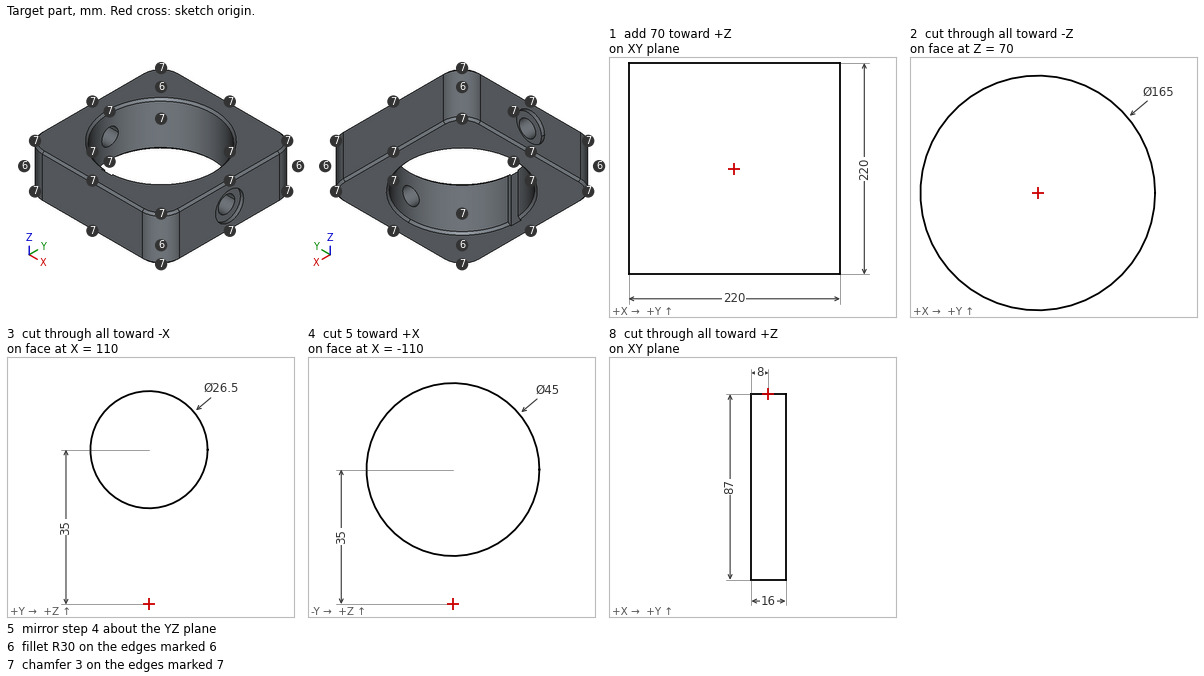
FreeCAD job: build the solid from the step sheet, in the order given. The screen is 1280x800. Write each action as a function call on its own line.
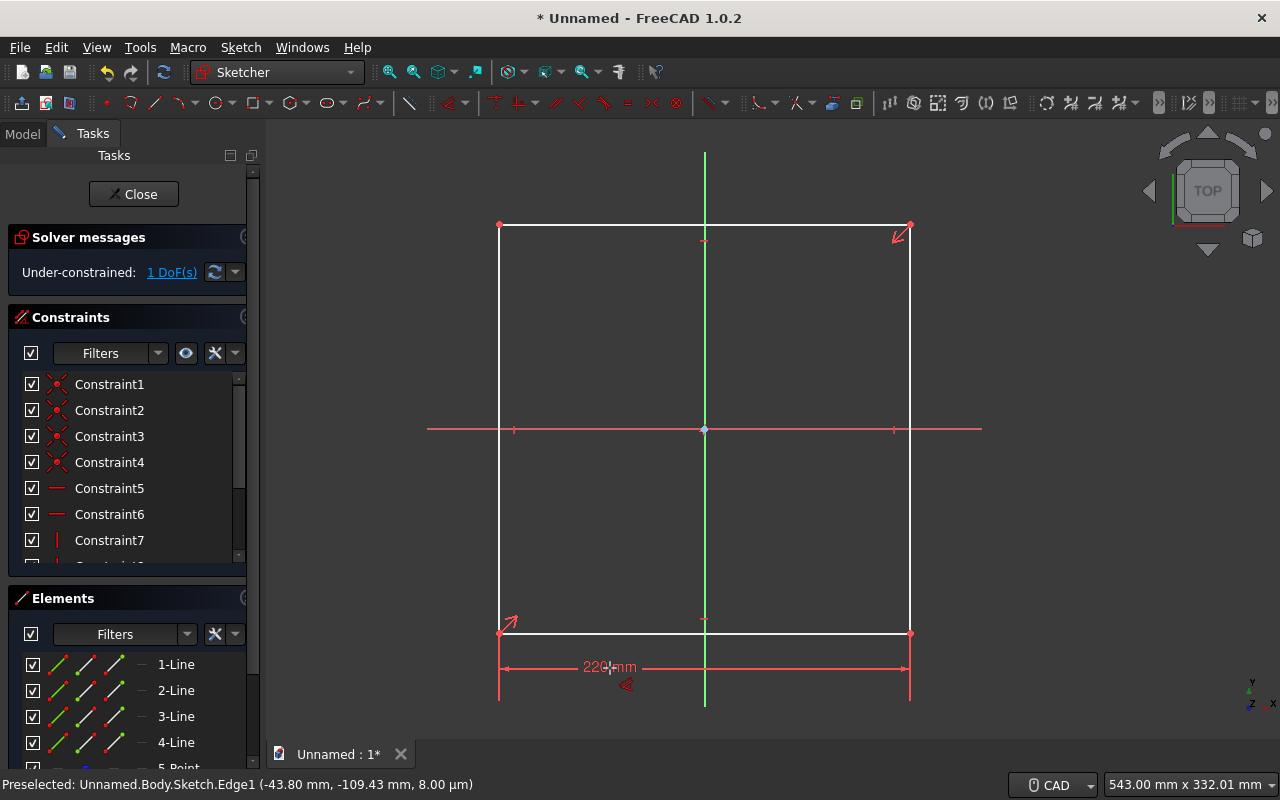
click(910, 511)
click(944, 335)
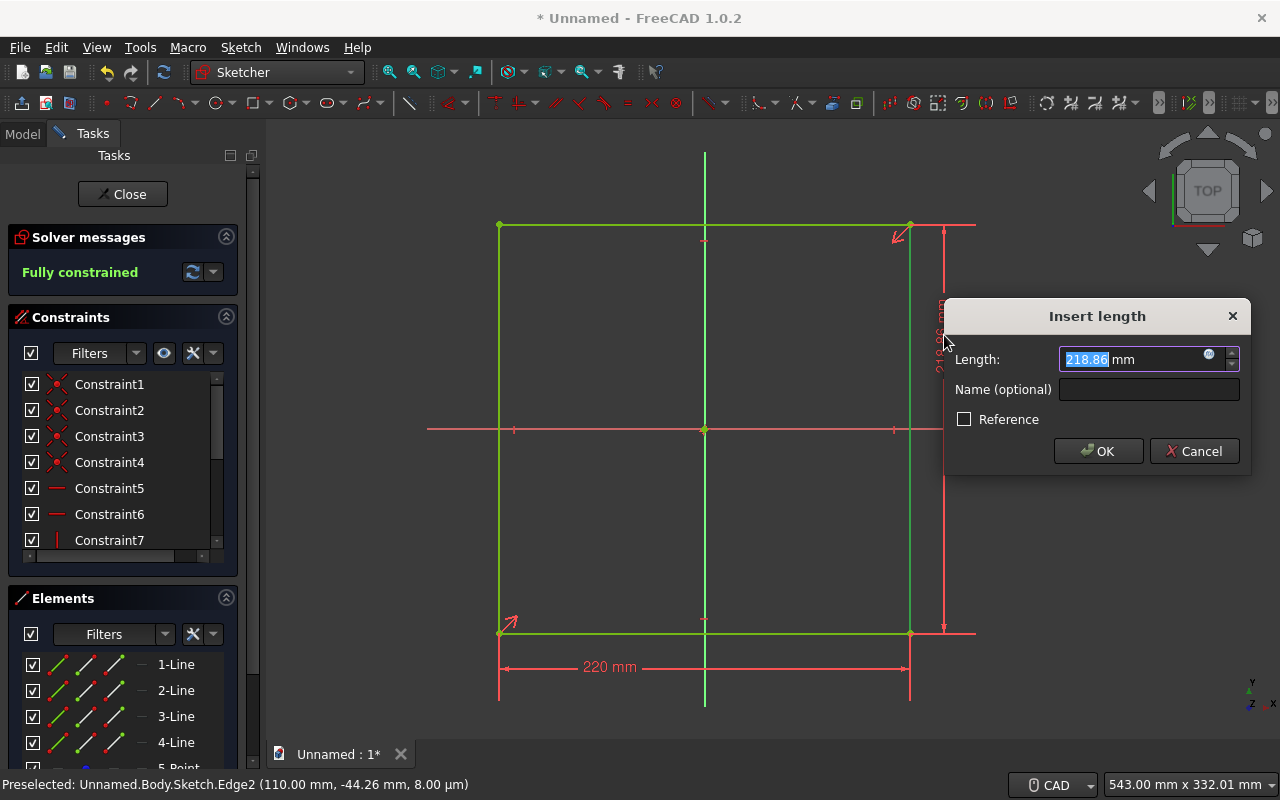
text(220)
key(Return)
key(Escape)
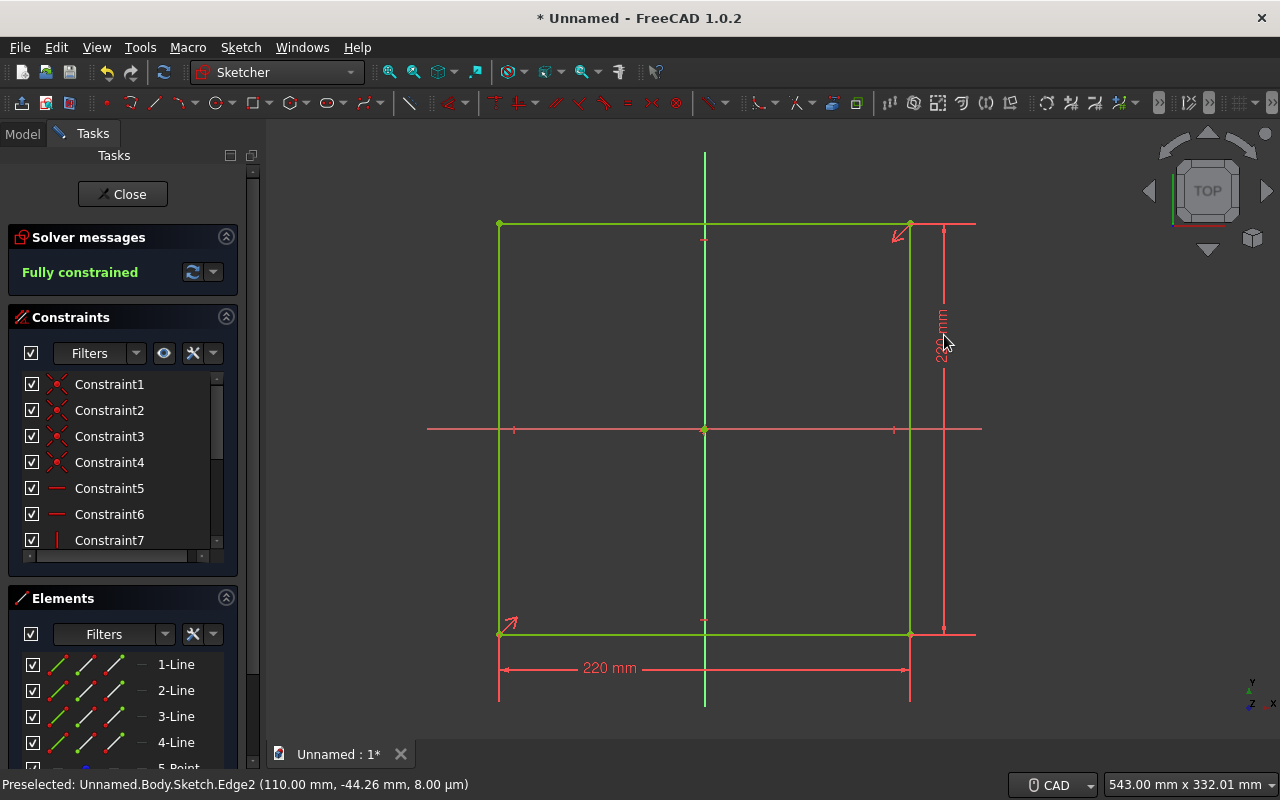
click(123, 194)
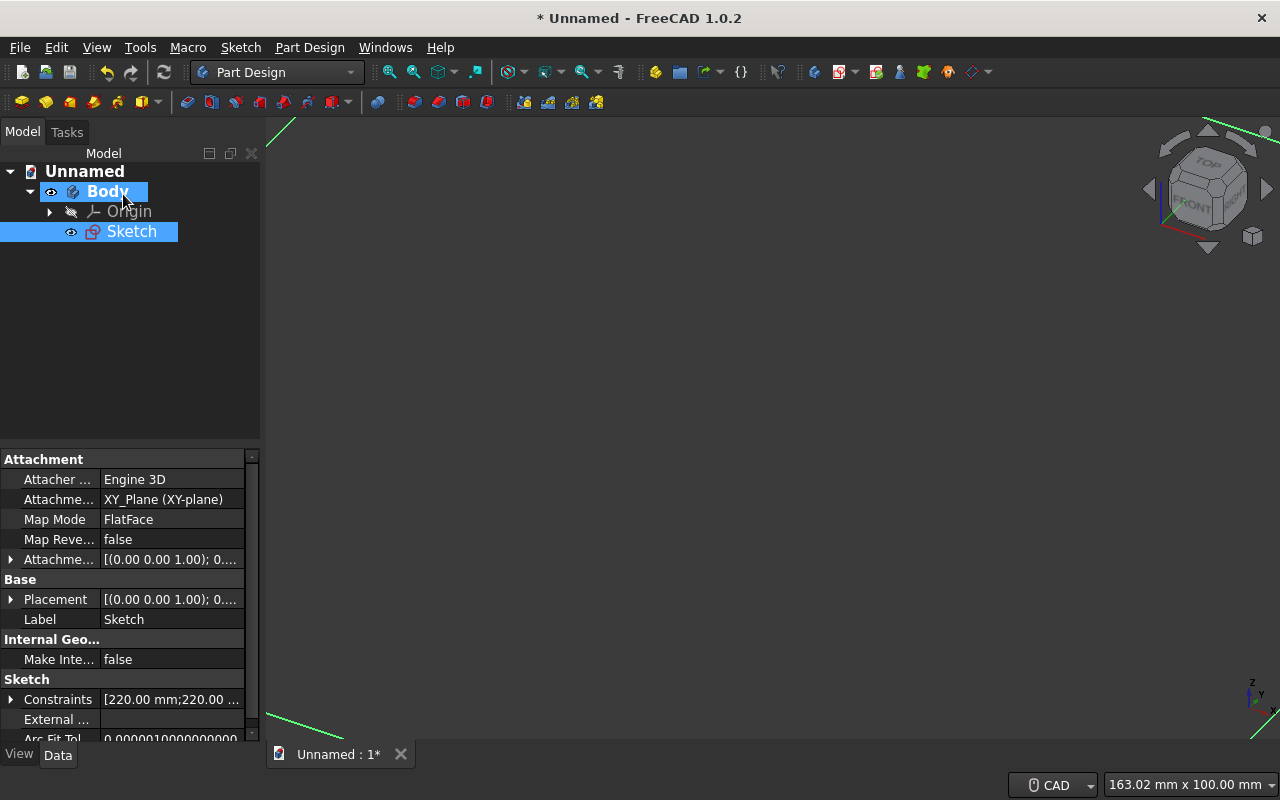
click(22, 102)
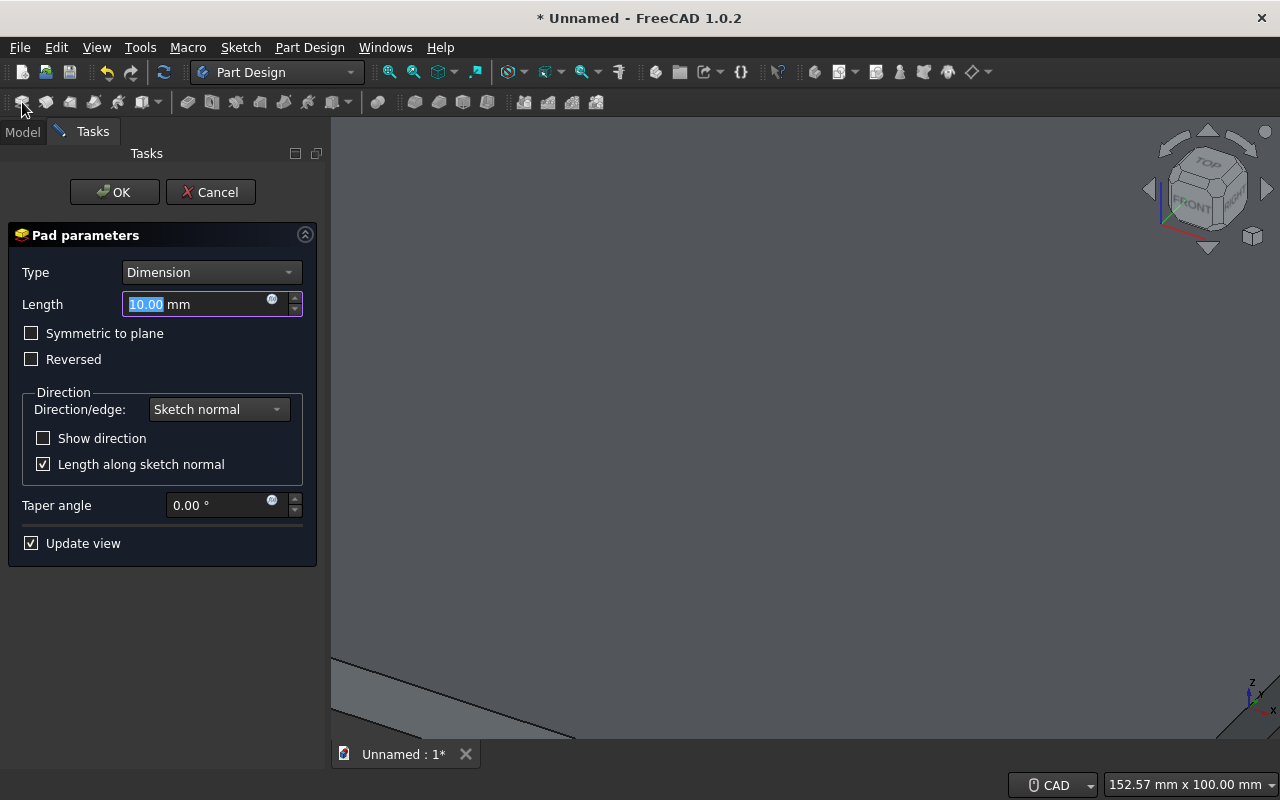
text(70)
key(Tab)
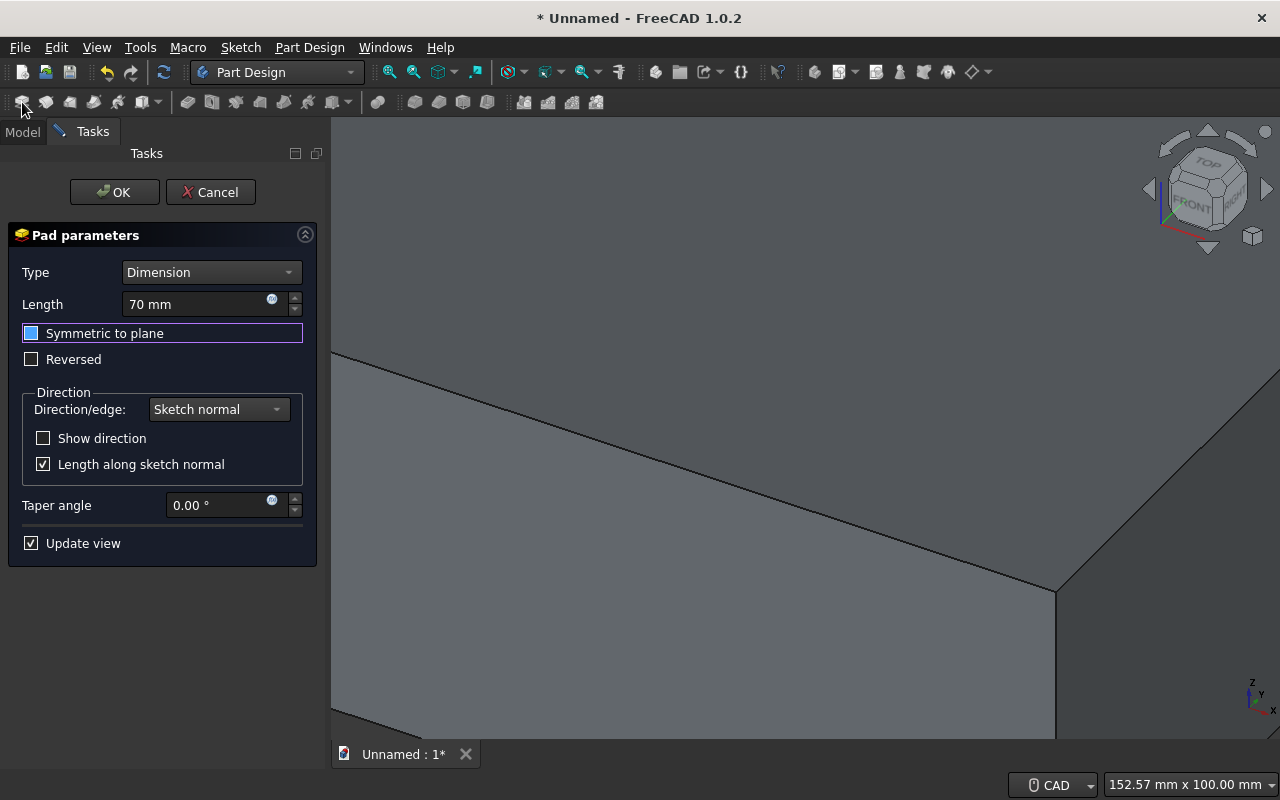
click(115, 192)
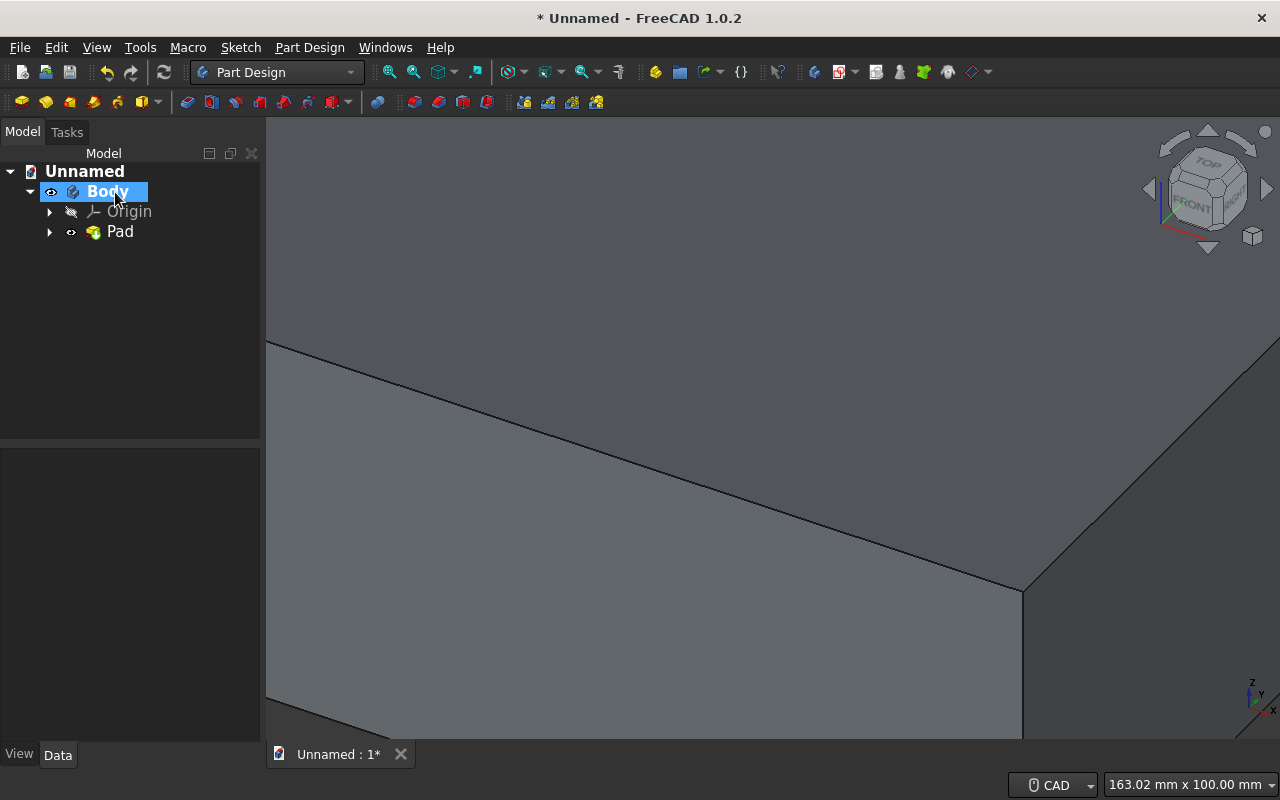
click(390, 72)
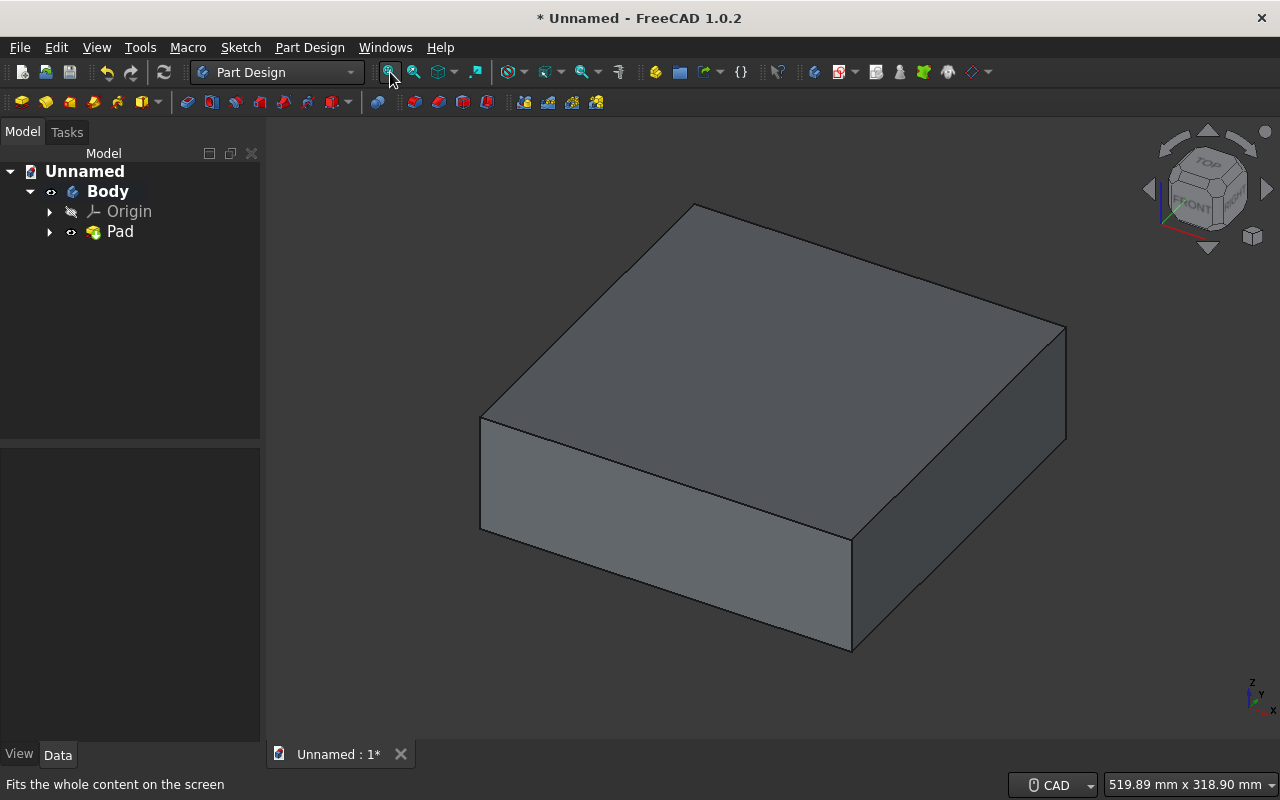
click(773, 371)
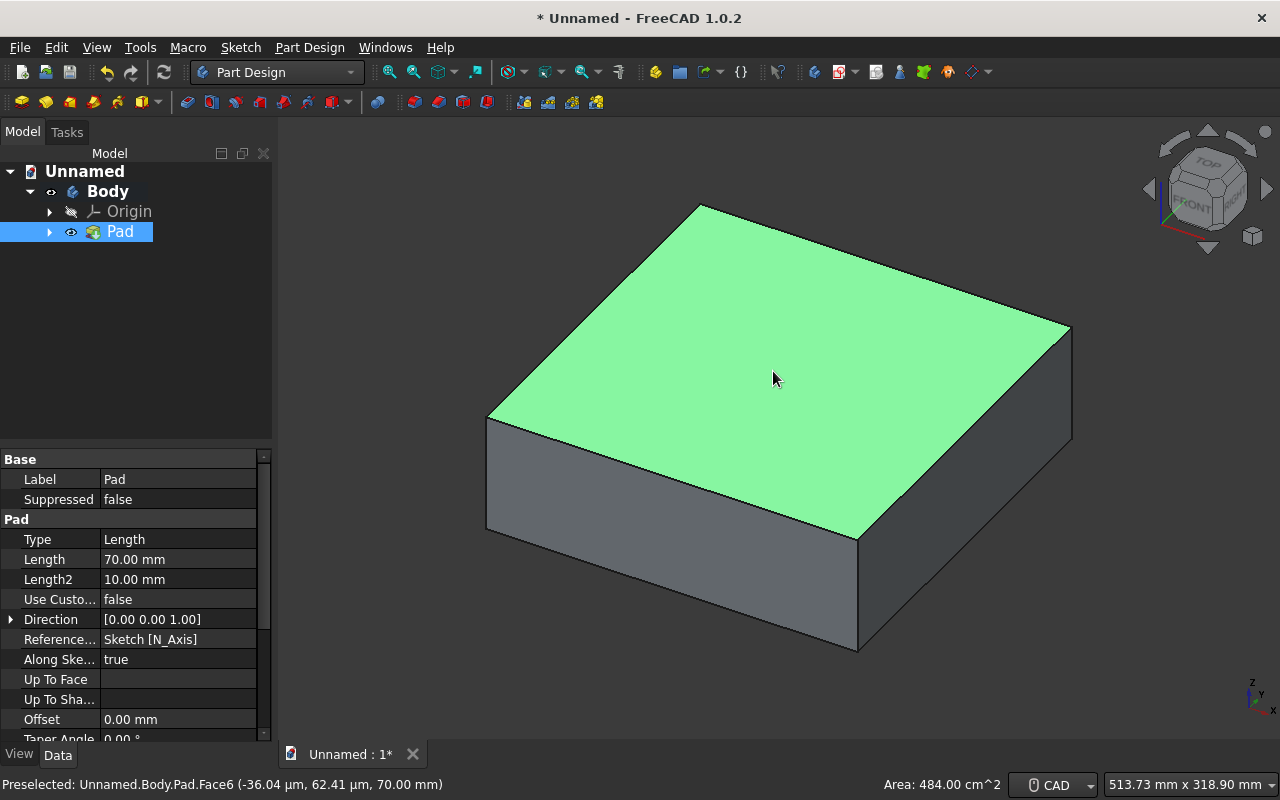
click(840, 72)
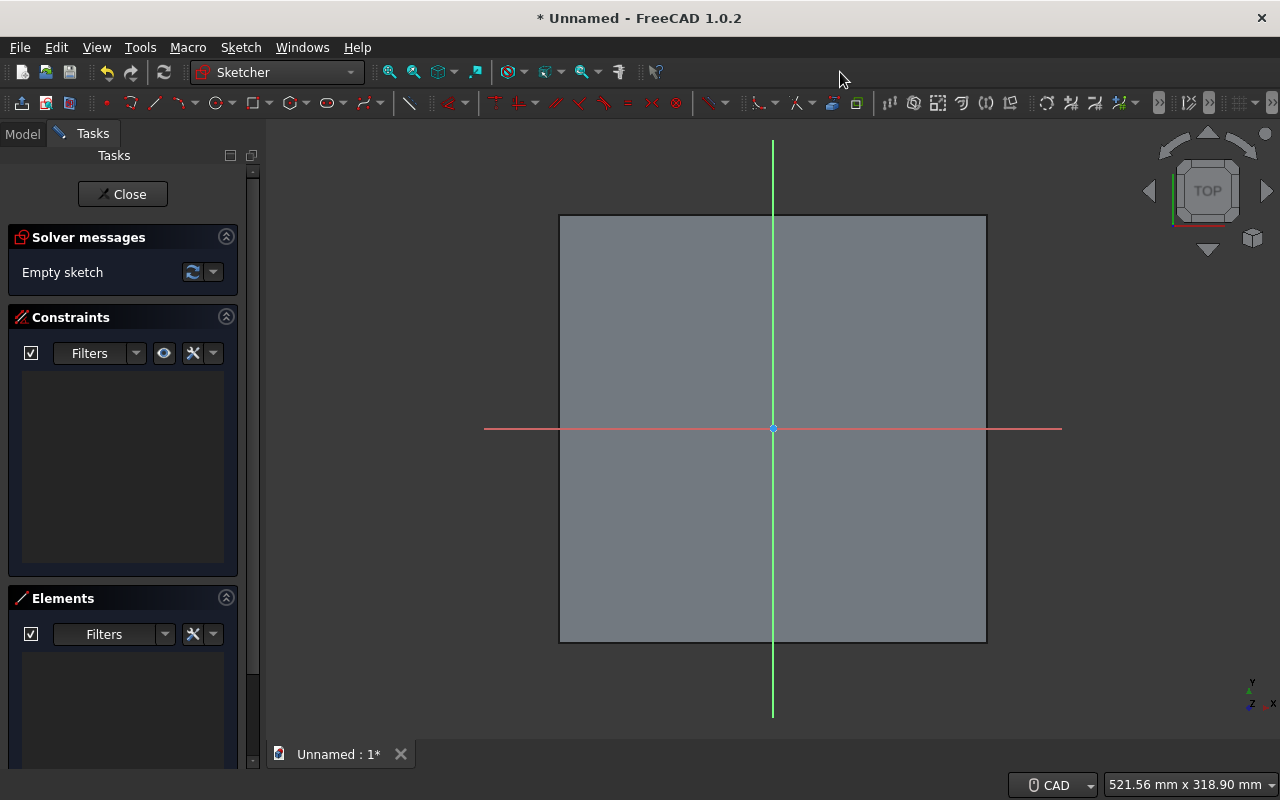
key(g)
key(c)